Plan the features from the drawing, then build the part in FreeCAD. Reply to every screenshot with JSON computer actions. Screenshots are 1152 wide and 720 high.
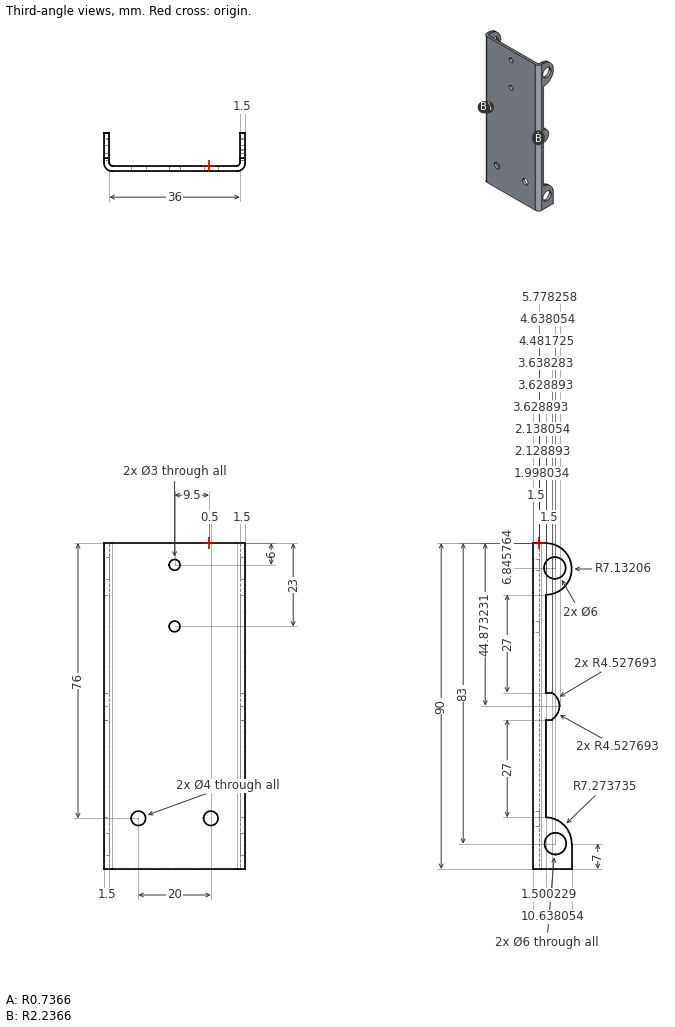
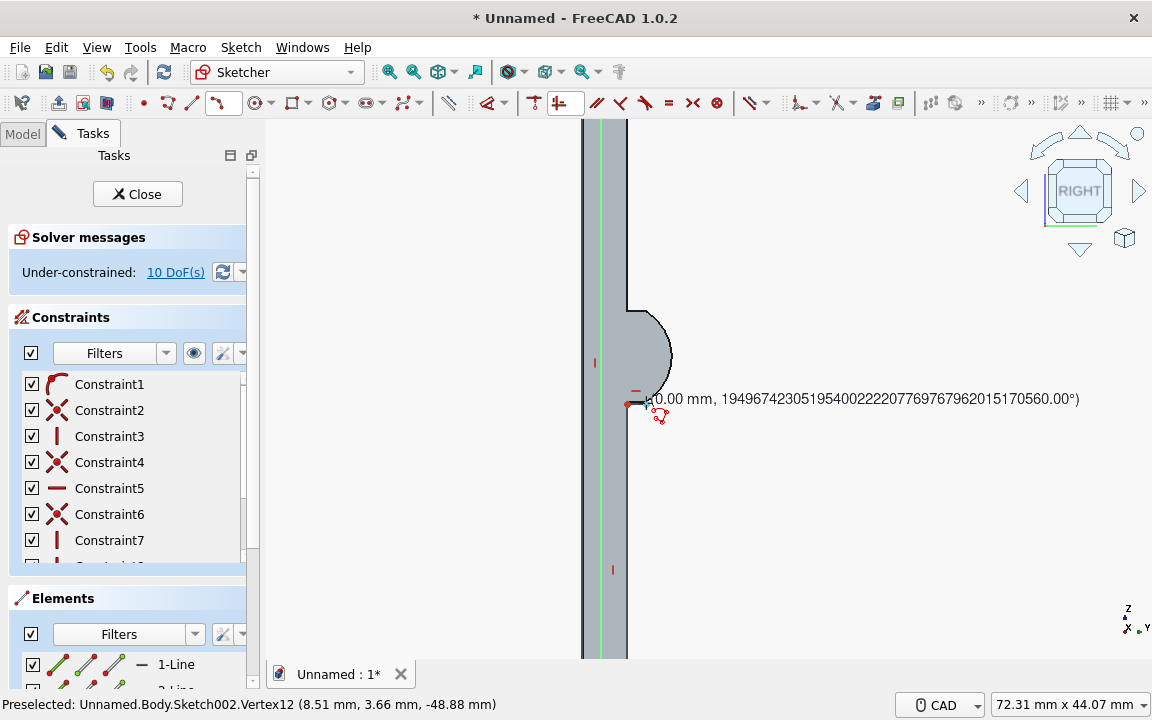
{"action": "left_click", "coordinate": [646, 311]}
{"action": "left_click", "coordinate": [627, 311]}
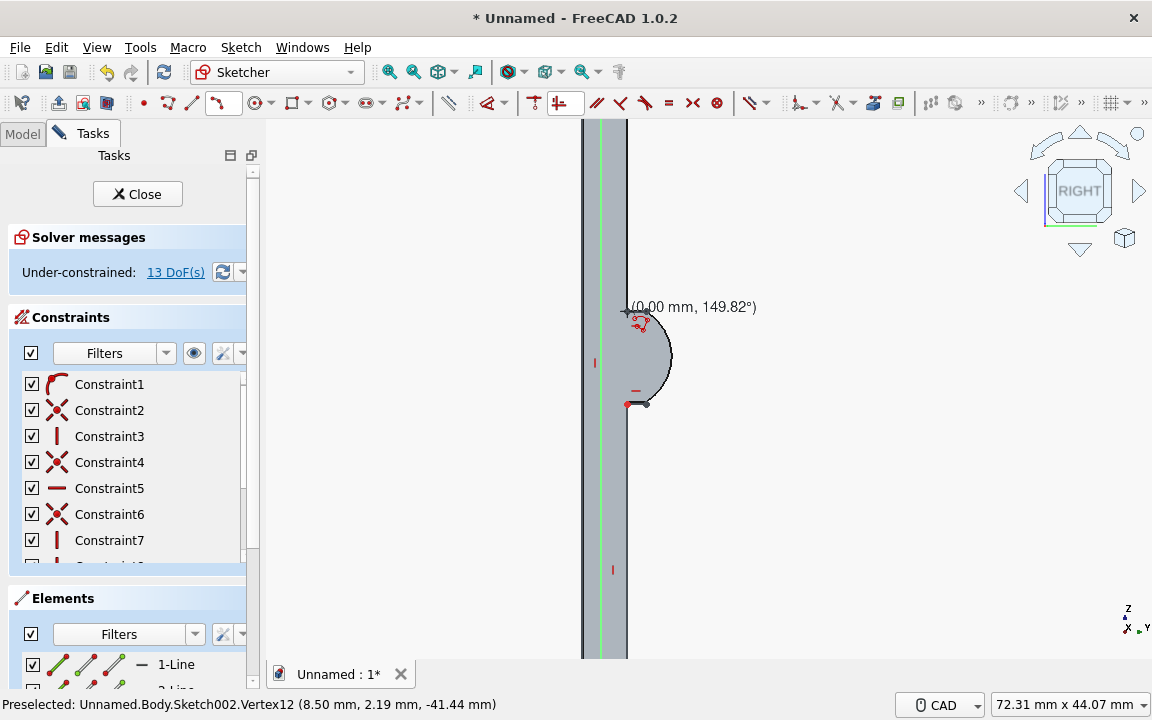
{"action": "scroll", "coordinate": [637, 403], "scroll_direction": "down", "scroll_amount": 6}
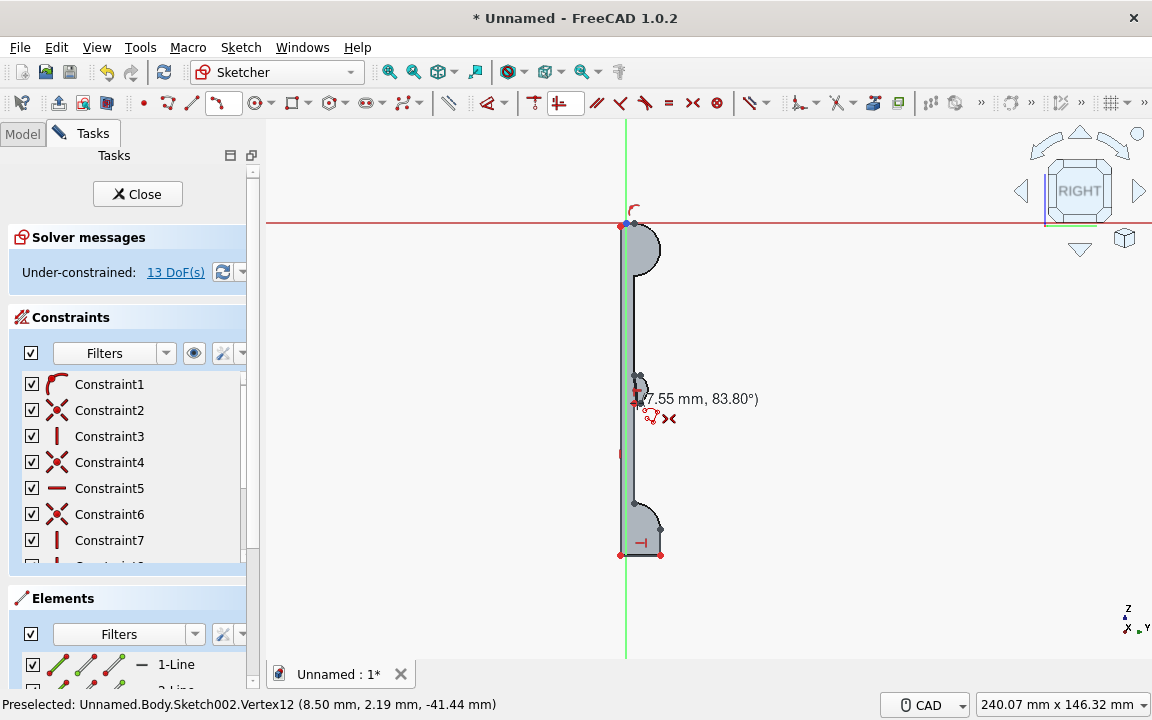
{"action": "scroll", "coordinate": [634, 276], "scroll_direction": "up", "scroll_amount": 4}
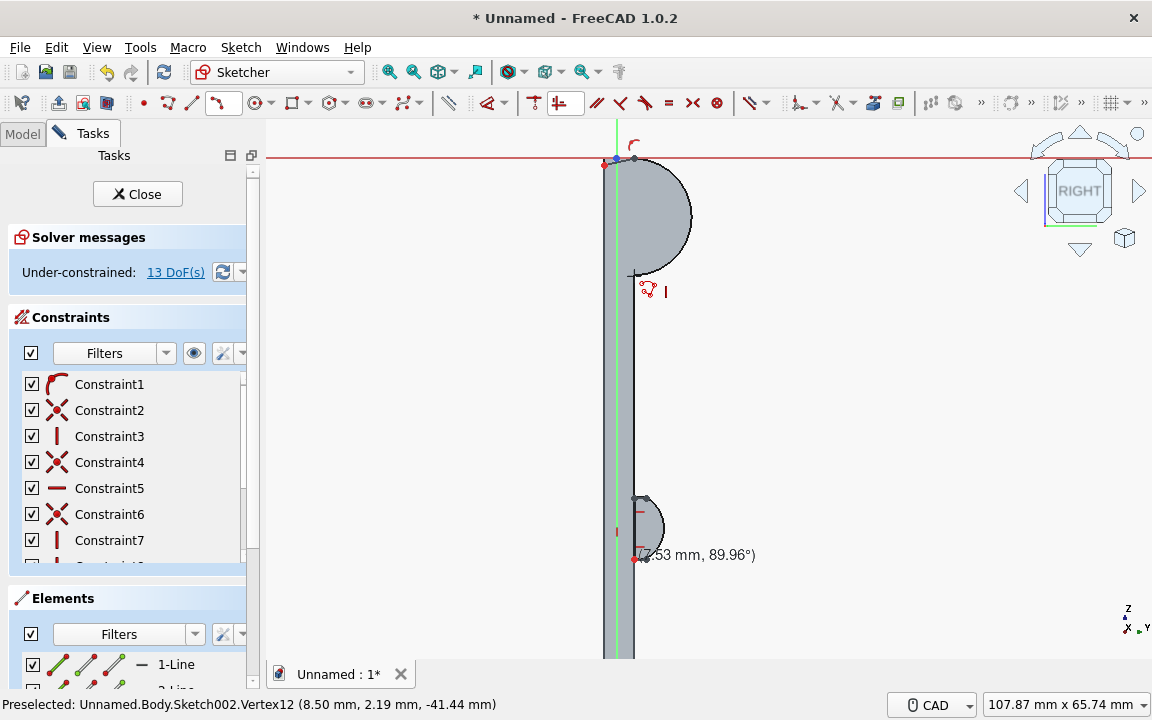
{"action": "left_click", "coordinate": [634, 276]}
{"action": "right_click", "coordinate": [634, 276]}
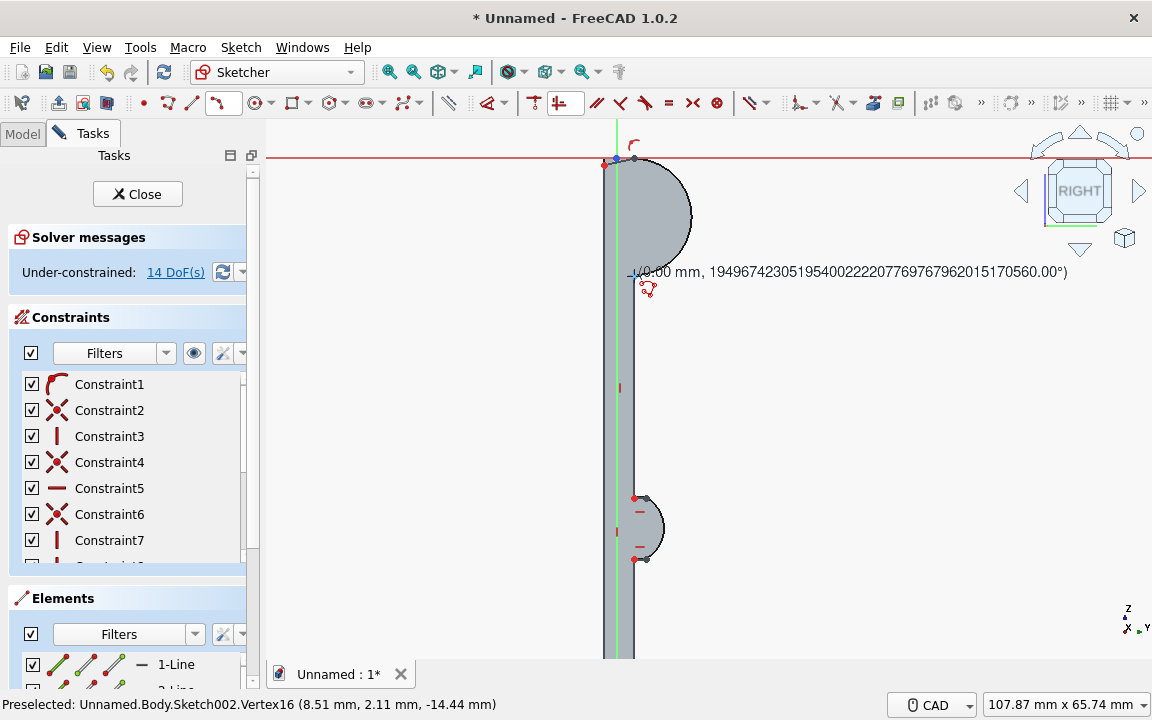
{"action": "key", "text": "g 3 a"}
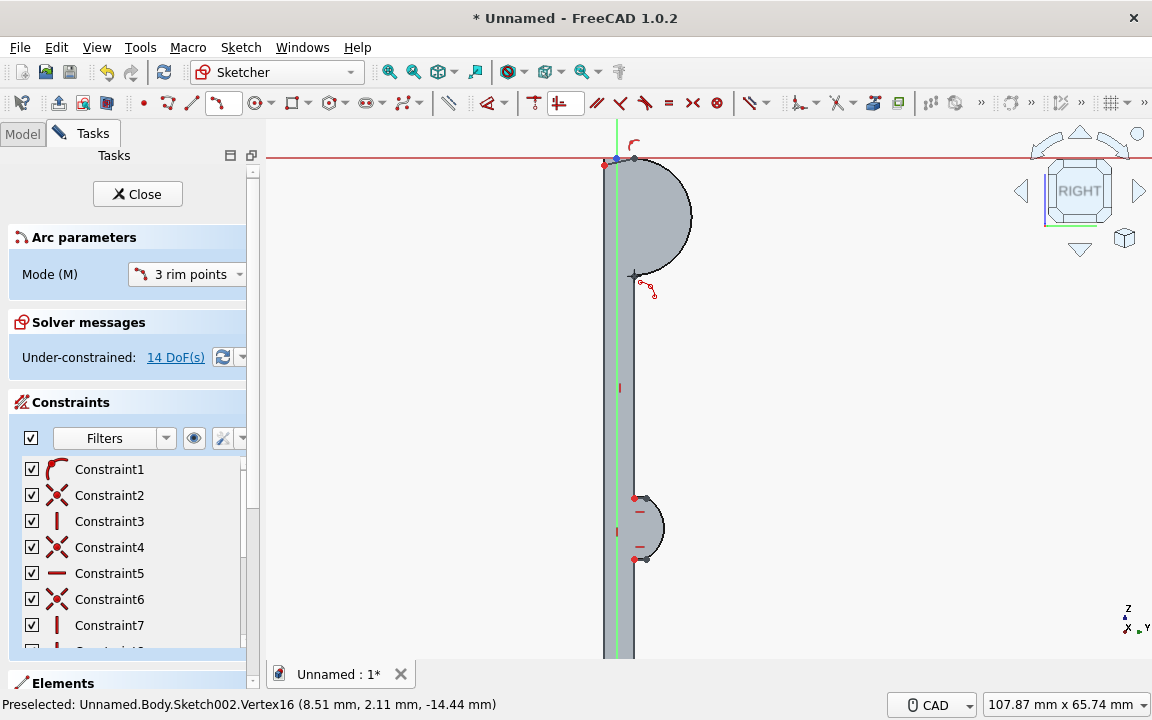
{"action": "scroll", "coordinate": [634, 276], "scroll_direction": "down", "scroll_amount": 4}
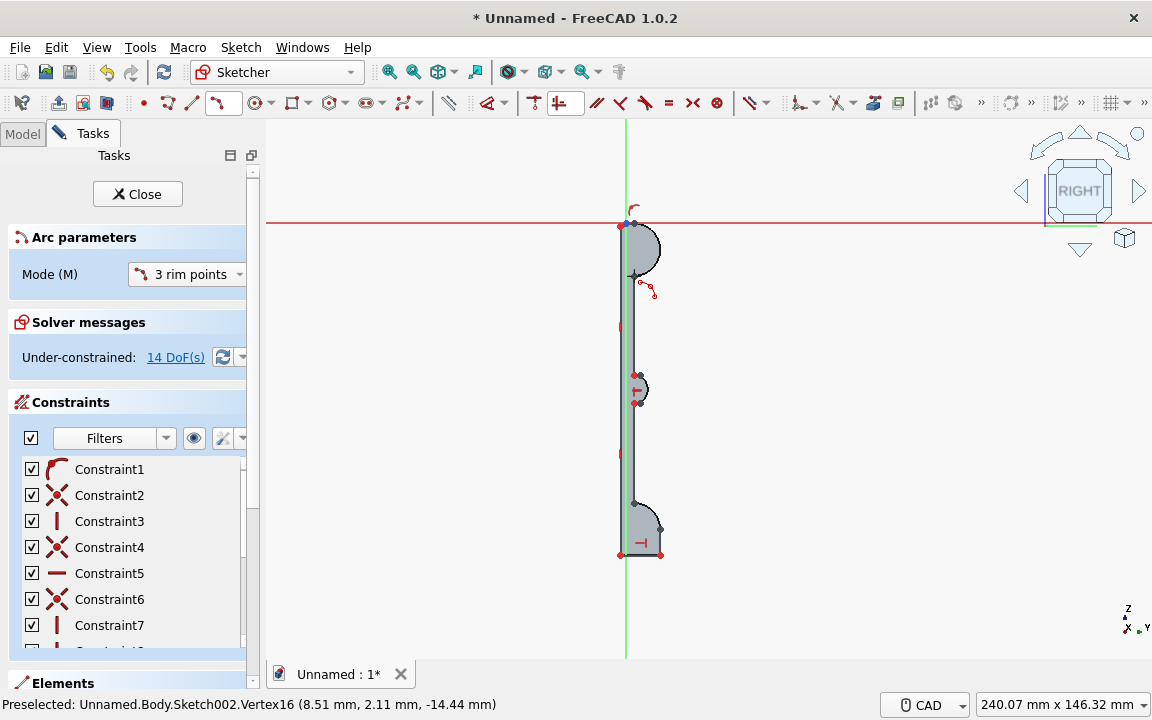
{"action": "scroll", "coordinate": [660, 530], "scroll_direction": "up", "scroll_amount": 2}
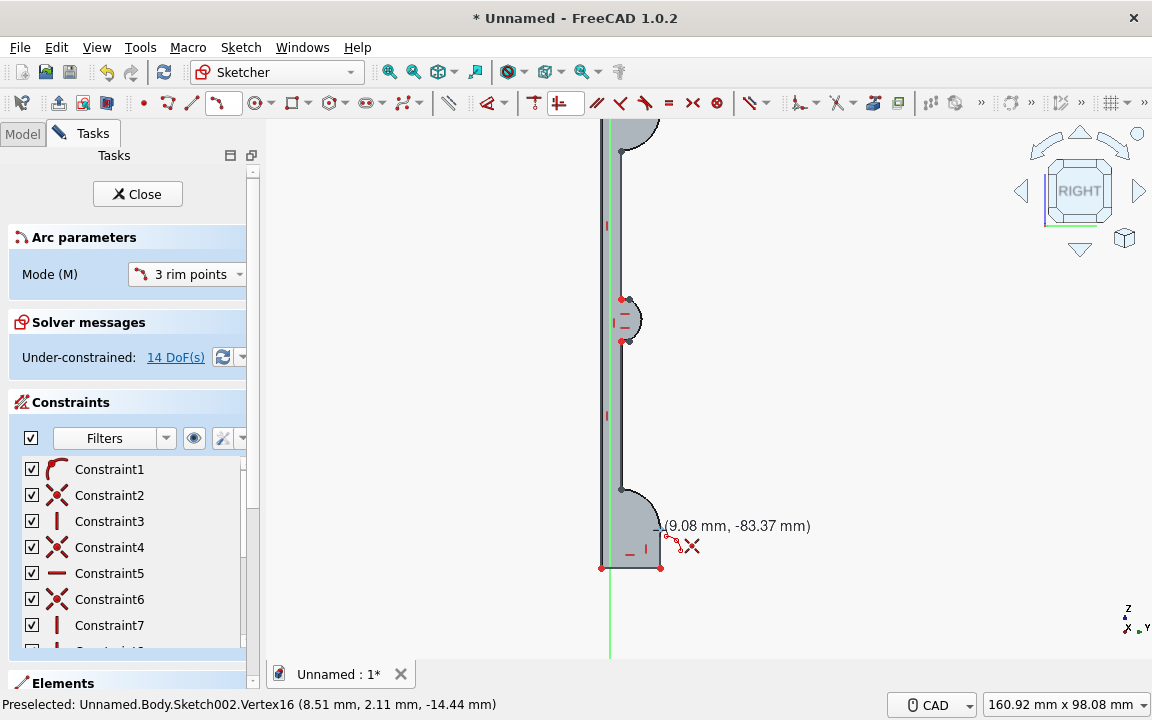
{"action": "left_click", "coordinate": [660, 530]}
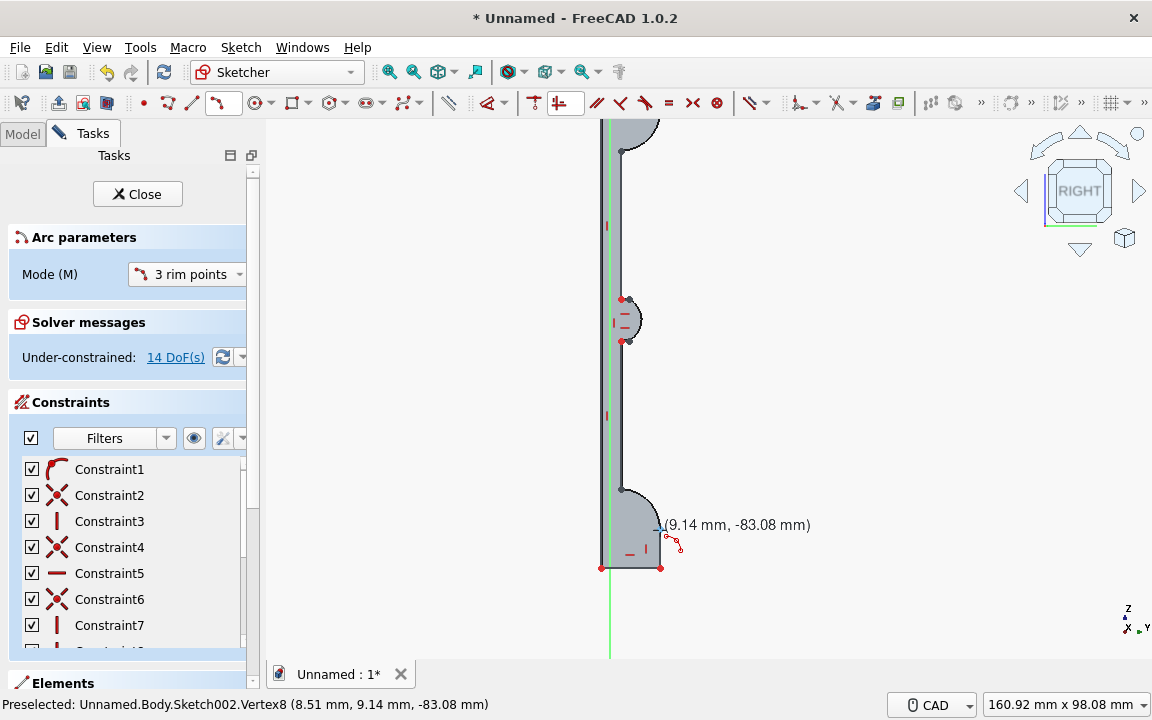
{"action": "scroll", "coordinate": [622, 489], "scroll_direction": "up", "scroll_amount": 2}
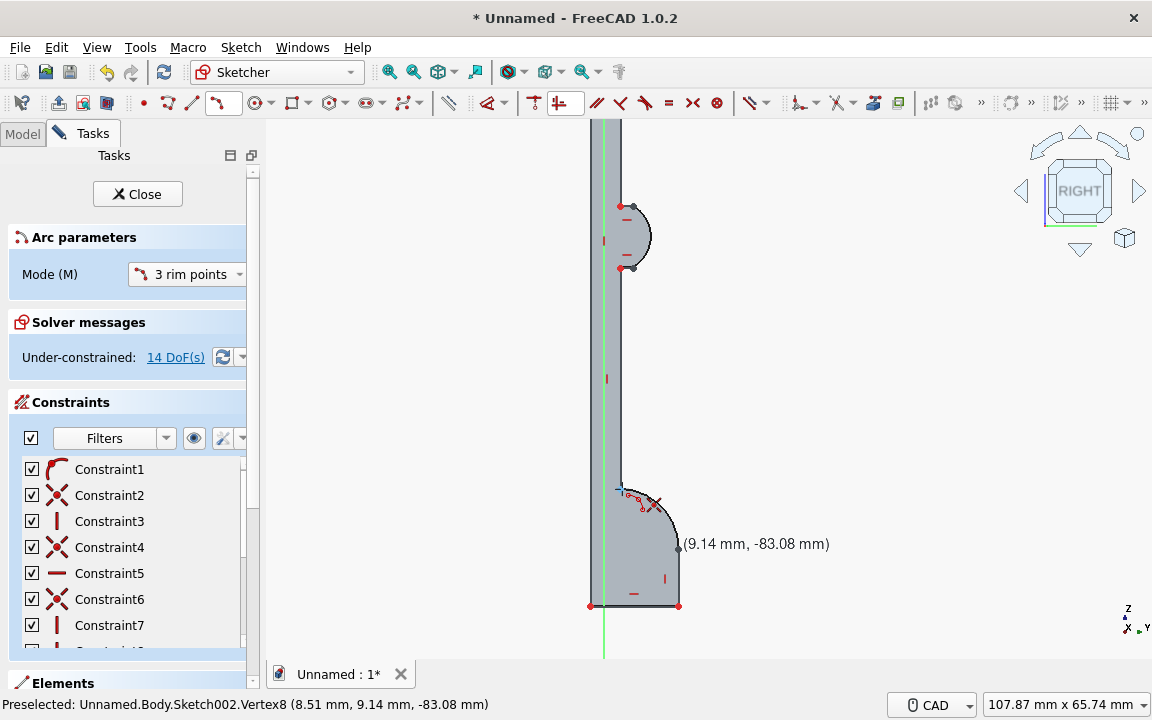
{"action": "left_click", "coordinate": [621, 490]}
{"action": "left_click", "coordinate": [662, 507]}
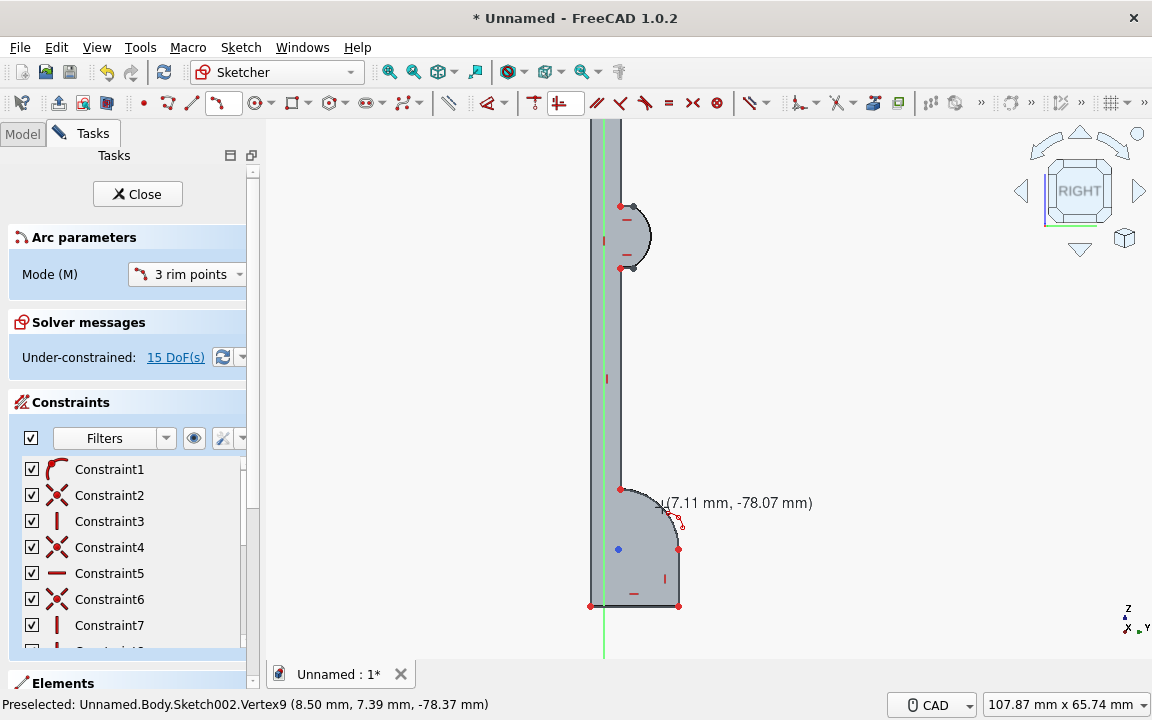
{"action": "scroll", "coordinate": [633, 267], "scroll_direction": "up", "scroll_amount": 5}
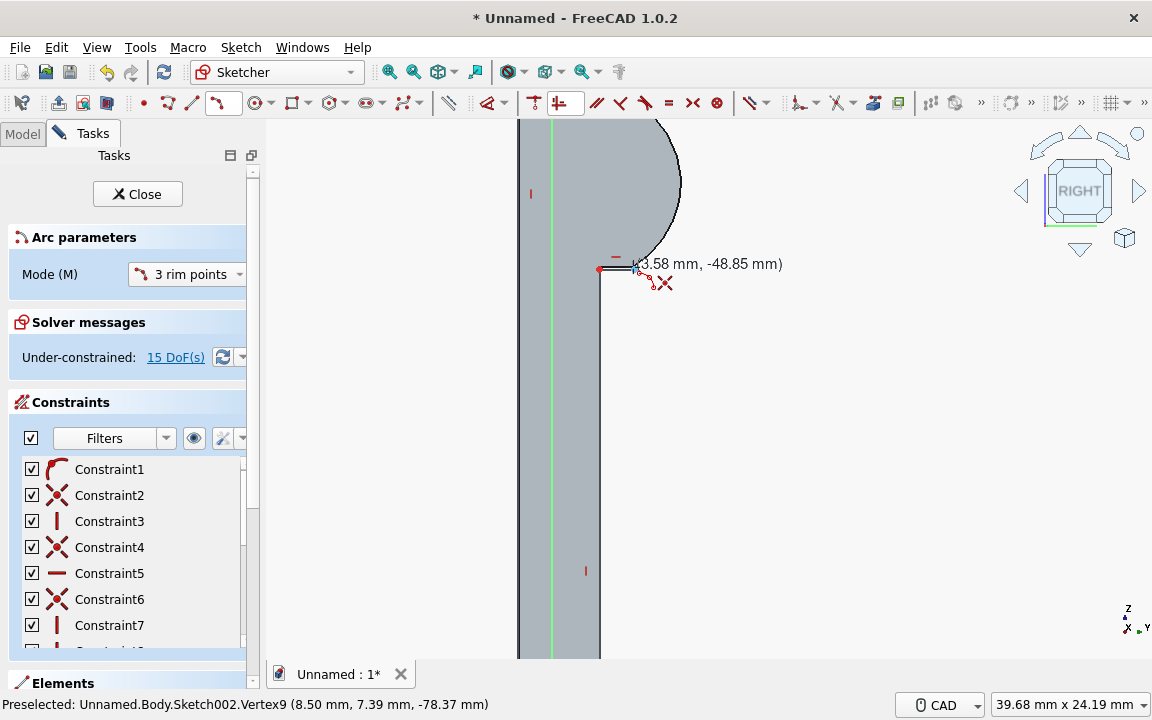
{"action": "left_click", "coordinate": [634, 270]}